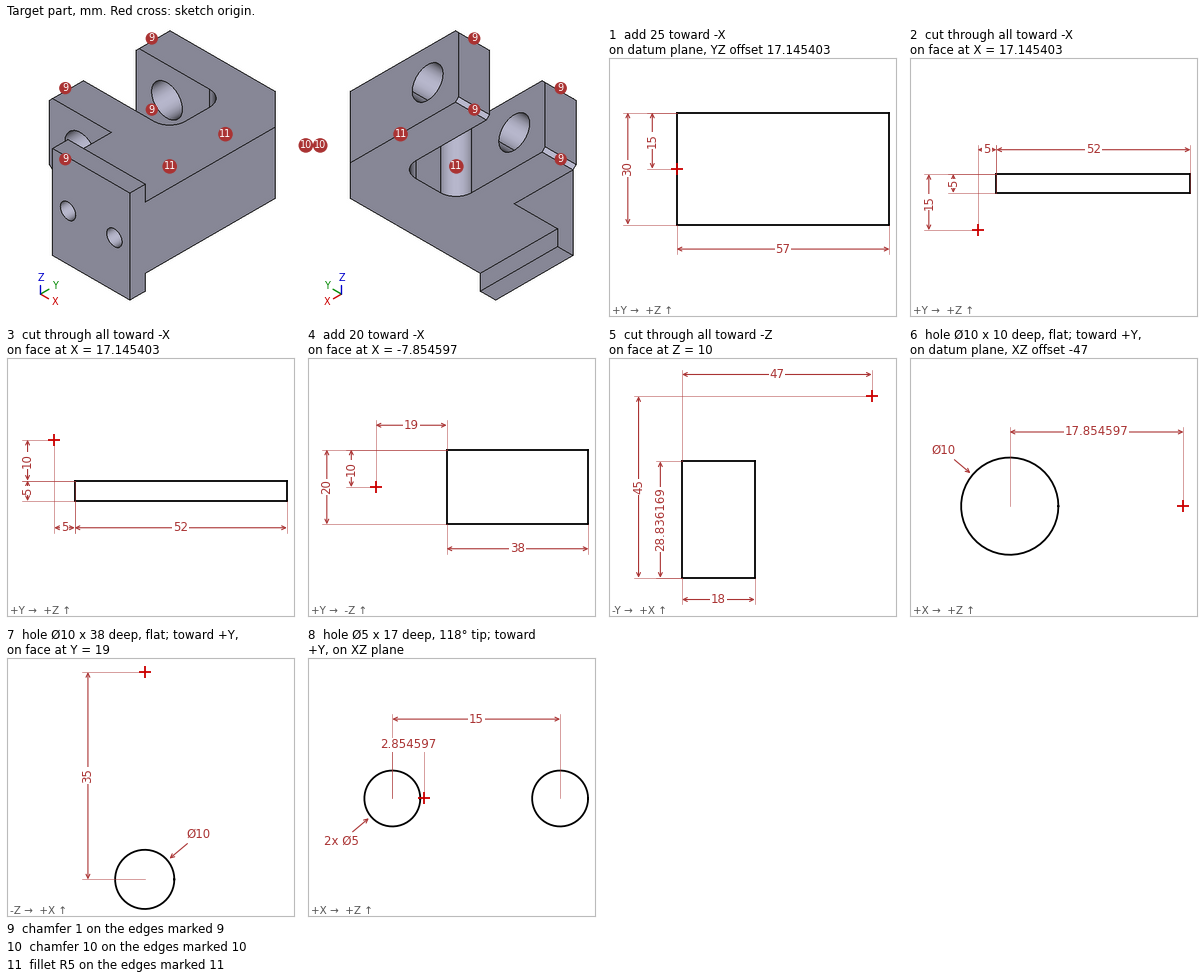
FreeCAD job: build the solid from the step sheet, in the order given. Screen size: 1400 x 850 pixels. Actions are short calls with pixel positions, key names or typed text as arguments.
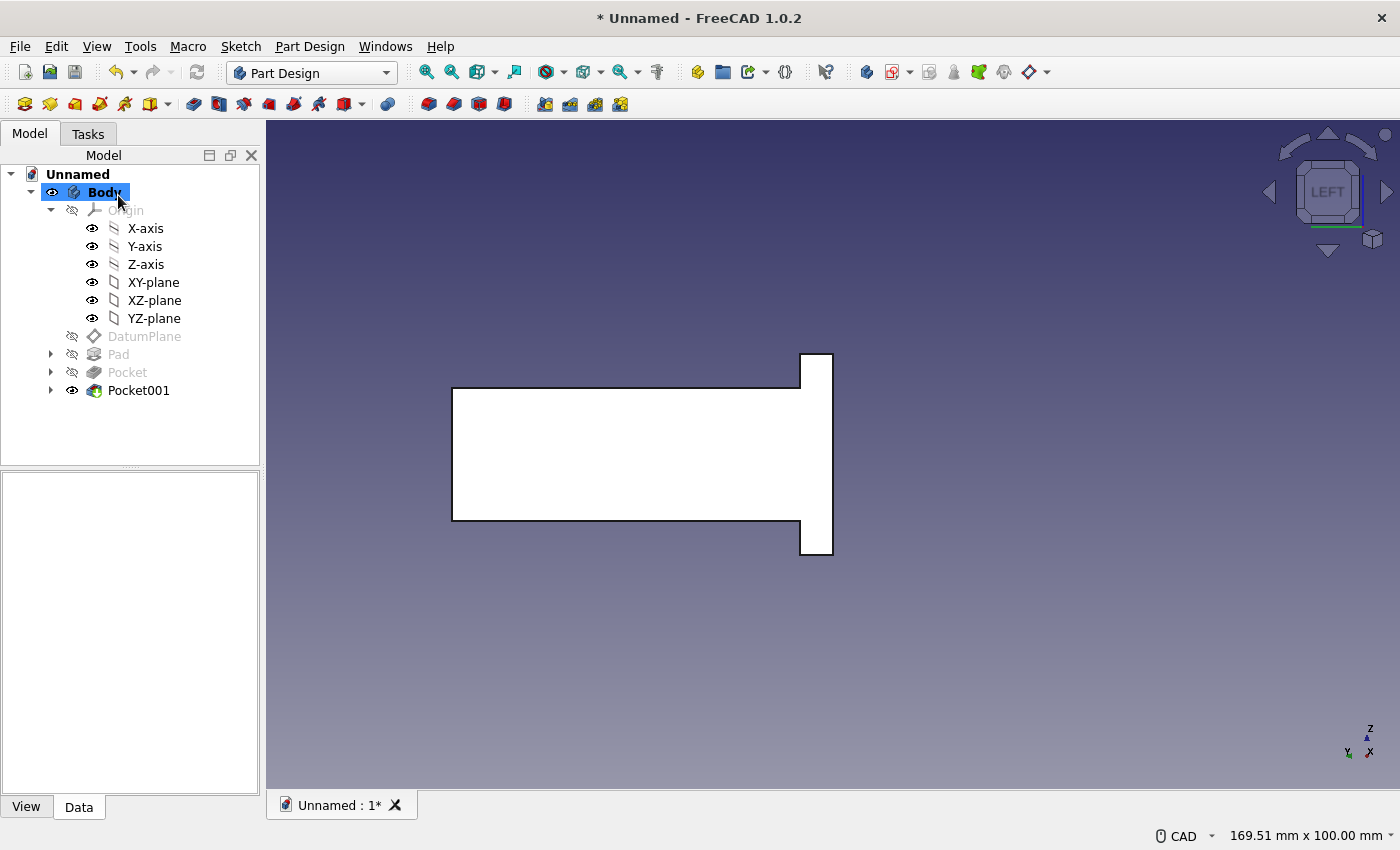
click(427, 72)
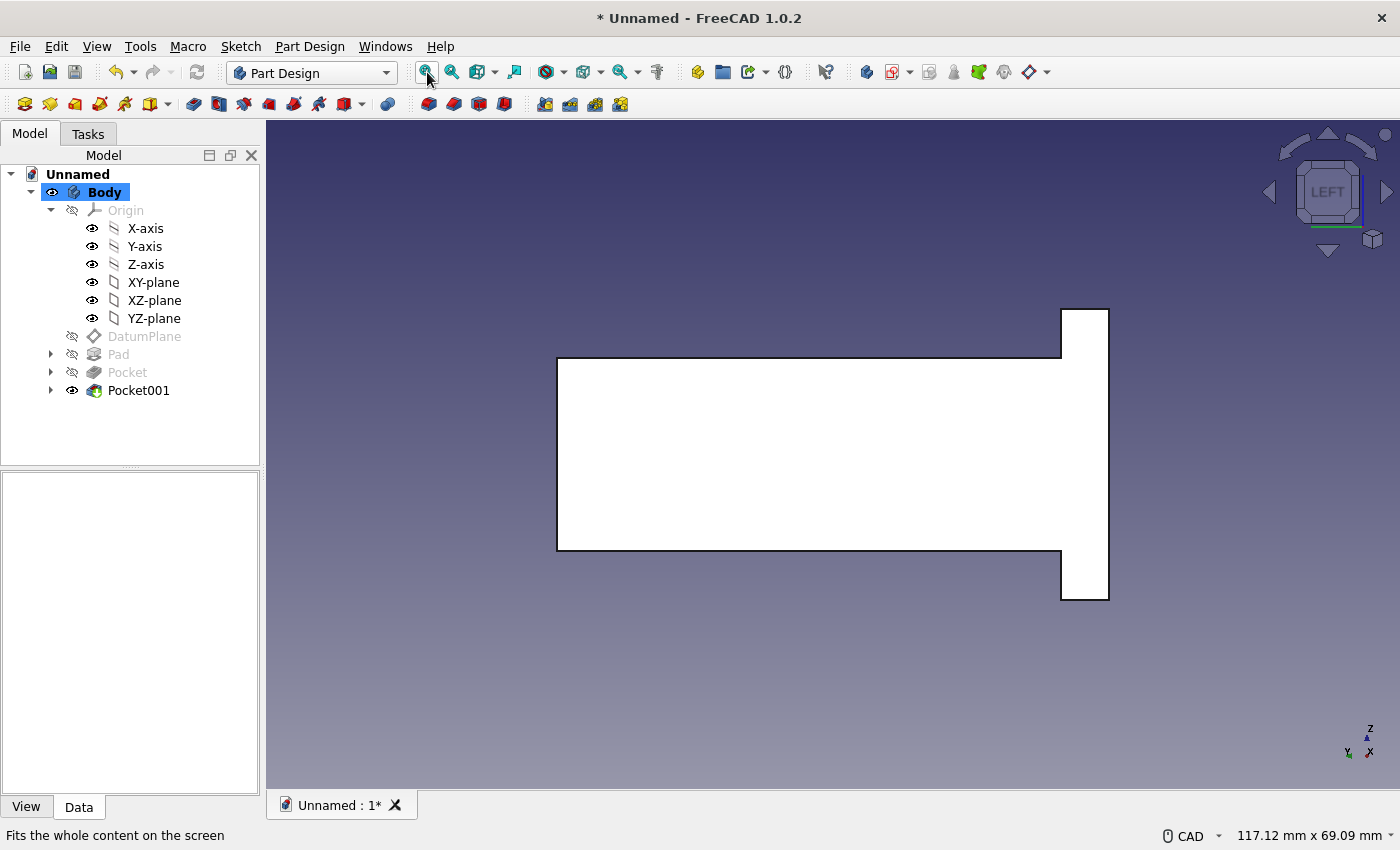
click(675, 453)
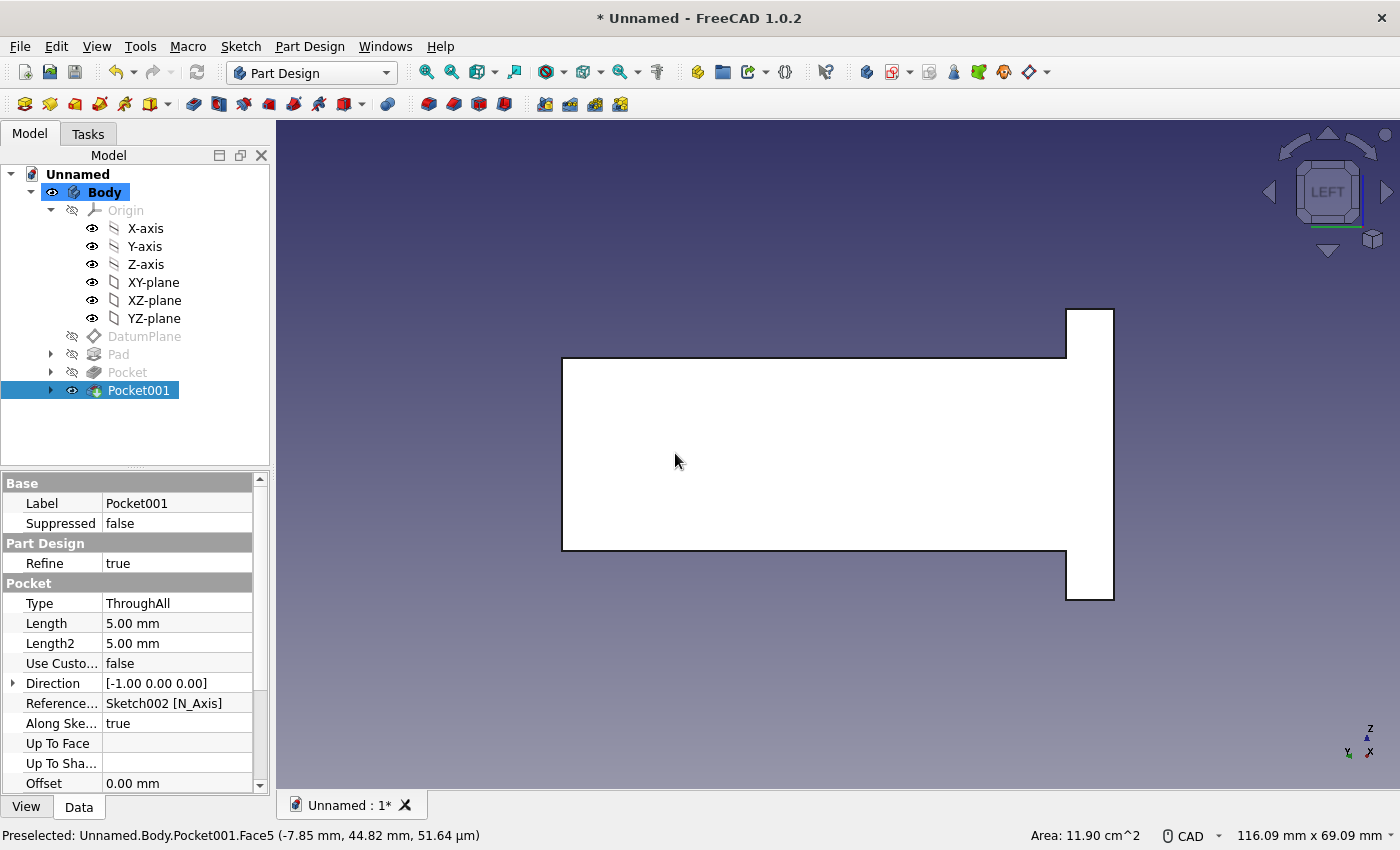
click(892, 72)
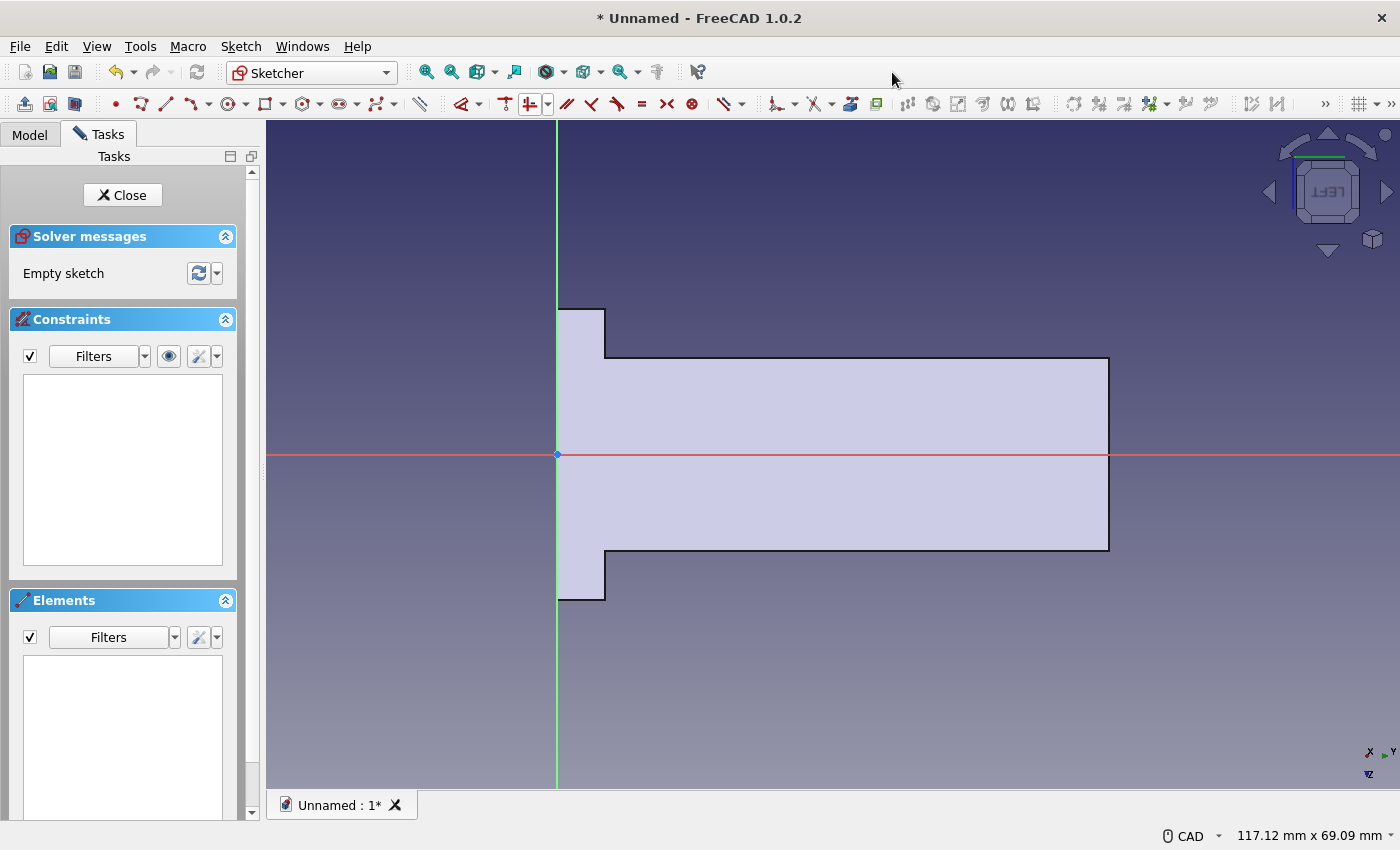
click(264, 104)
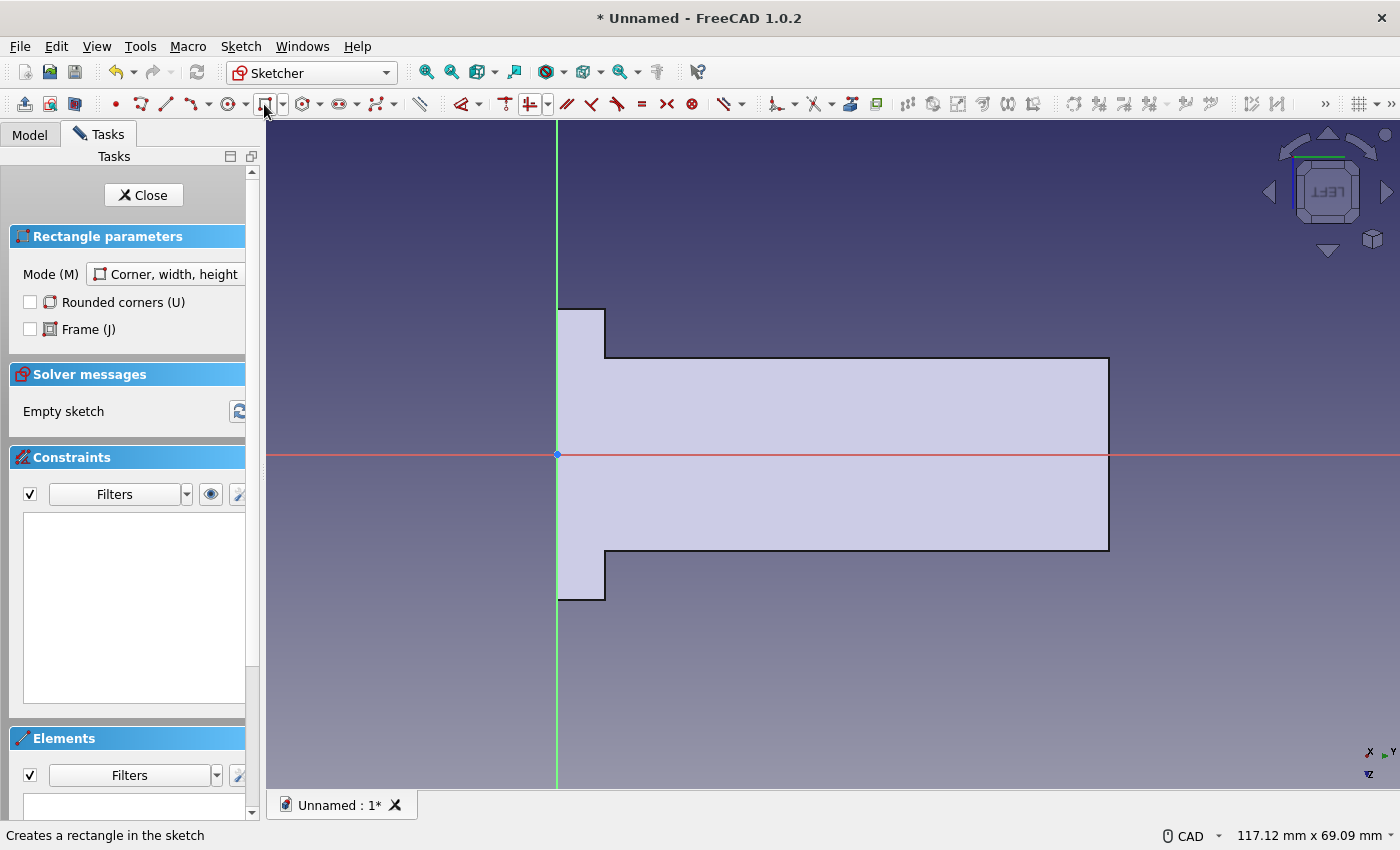
click(741, 358)
click(1109, 551)
key(Escape)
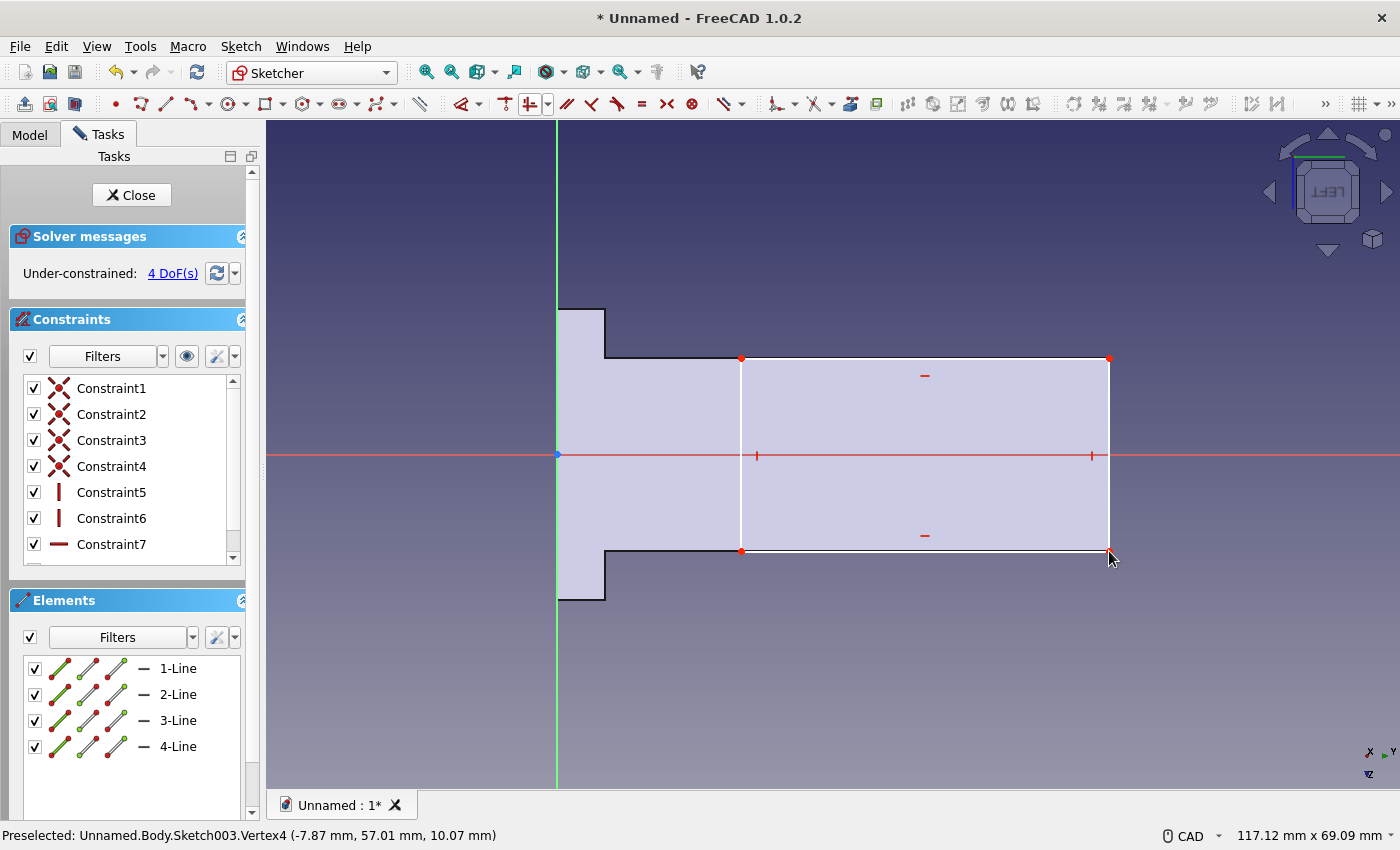
click(460, 104)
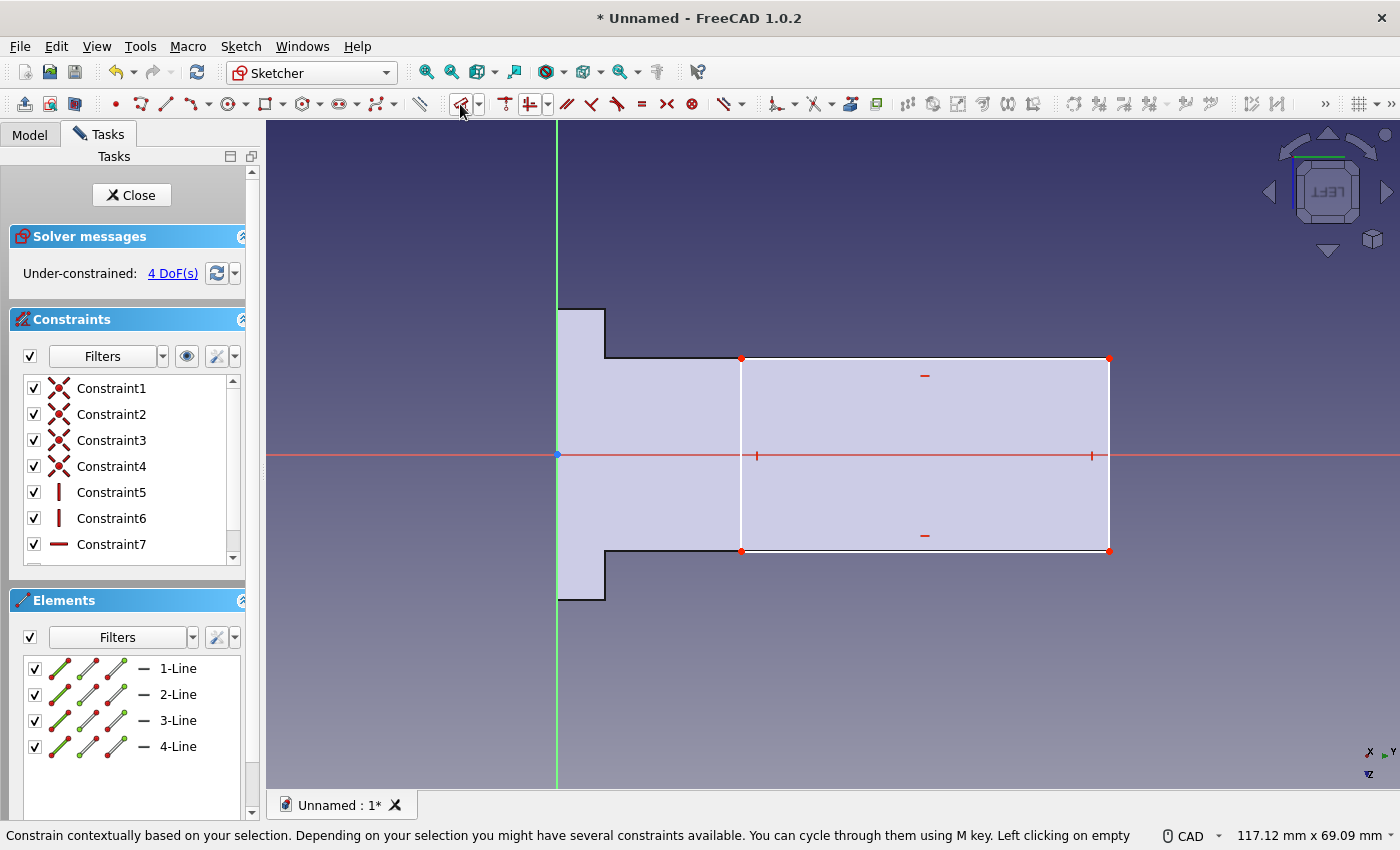
click(741, 417)
click(707, 411)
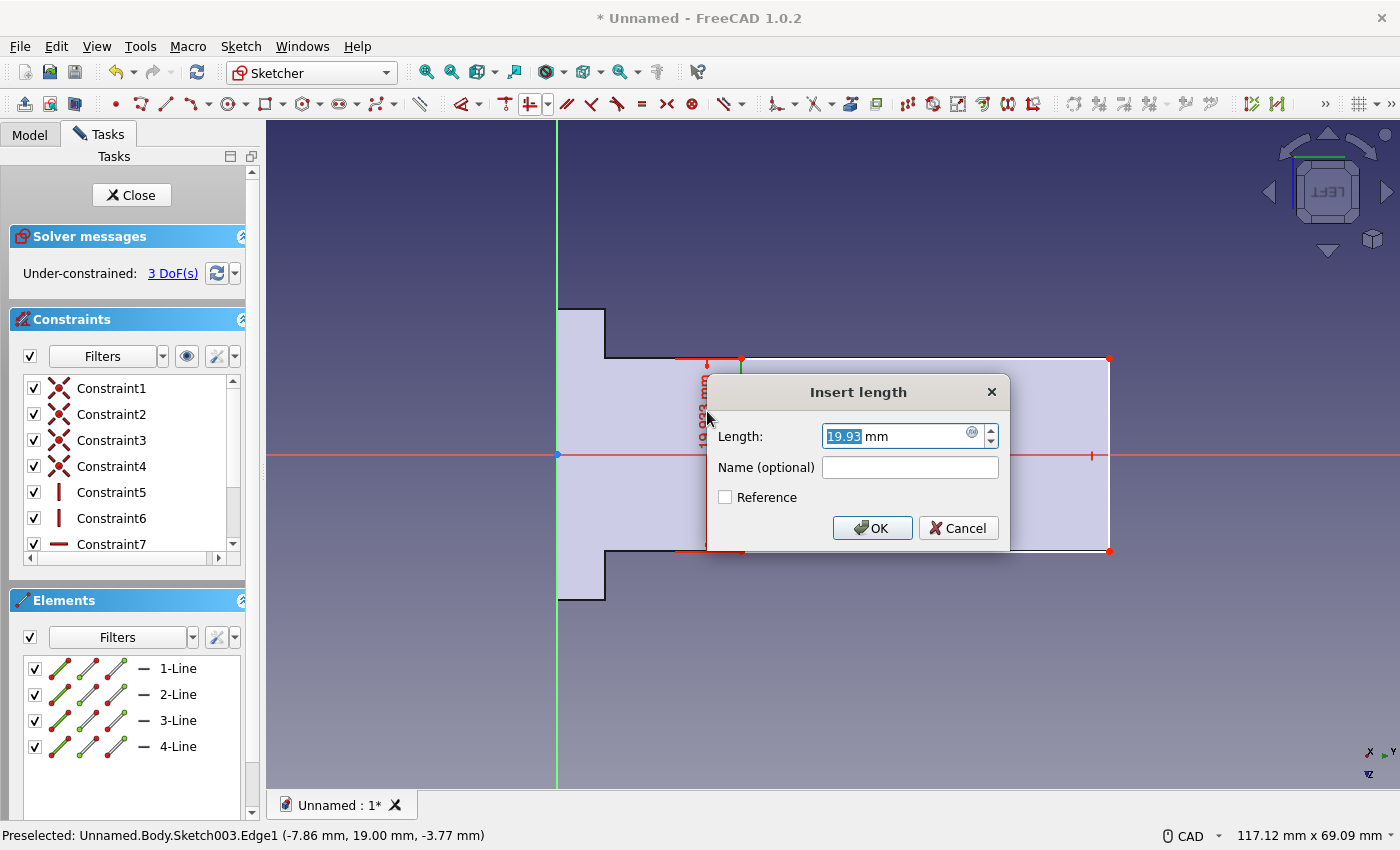
text(20)
key(Return)